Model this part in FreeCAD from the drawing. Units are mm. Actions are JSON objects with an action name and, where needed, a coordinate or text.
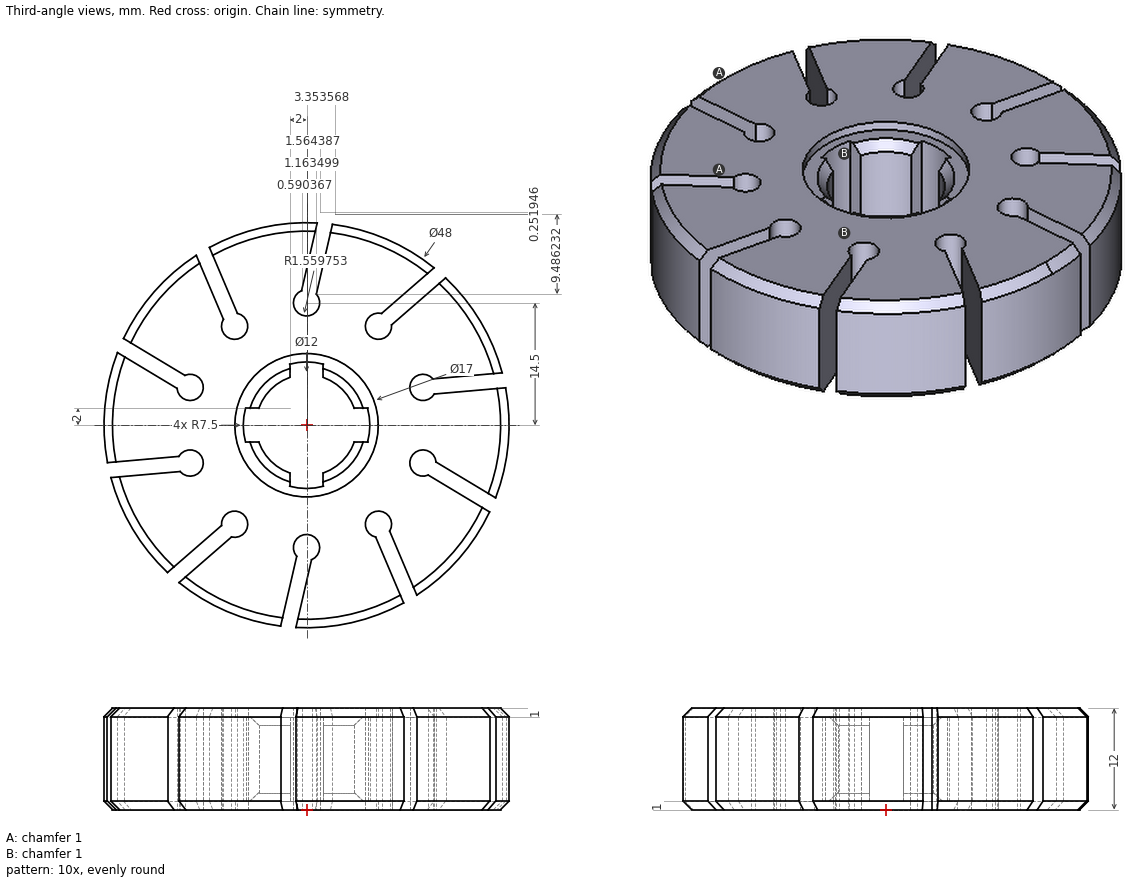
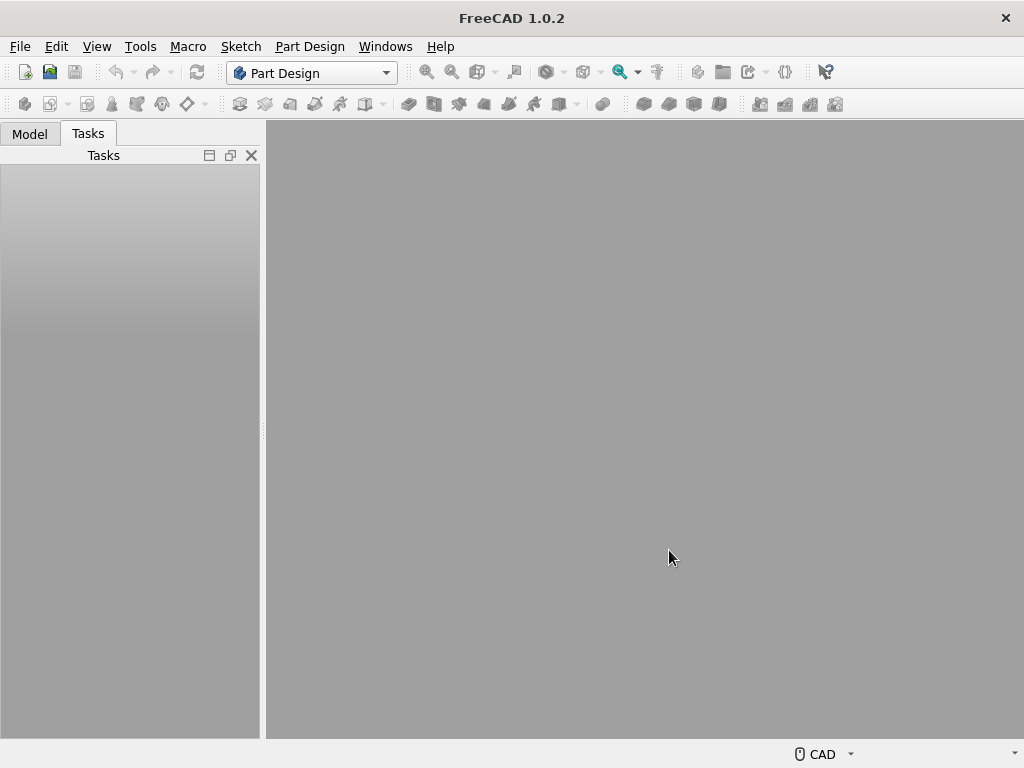
{"action": "left_click", "coordinate": [25, 72]}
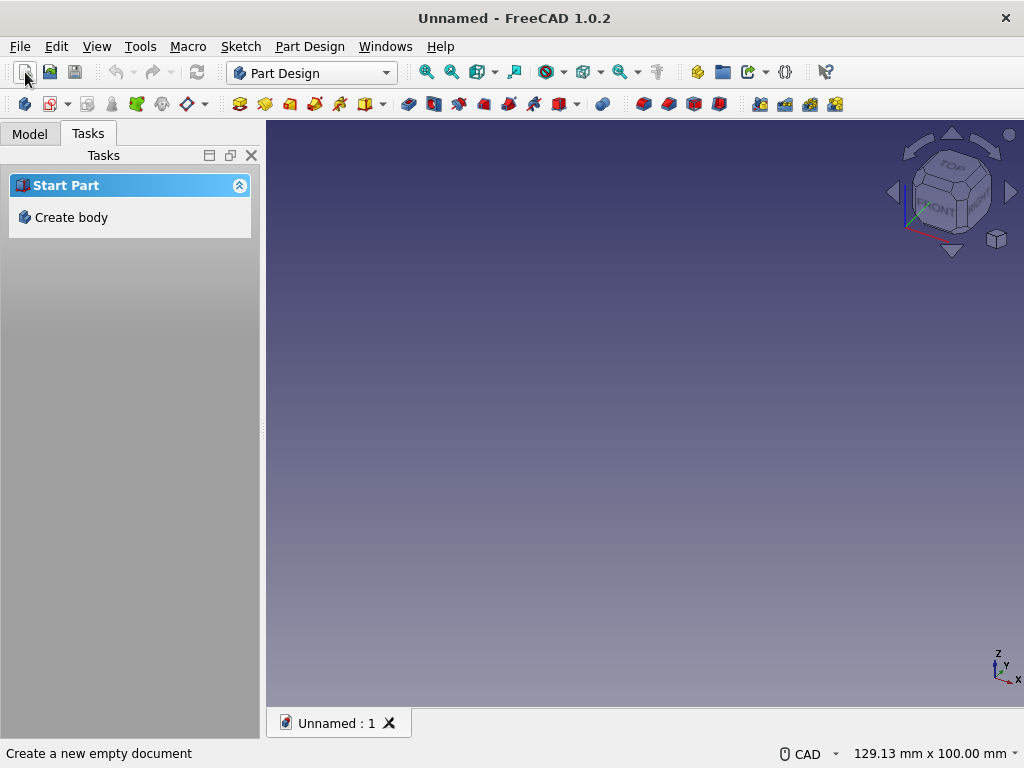
{"action": "left_click", "coordinate": [50, 104]}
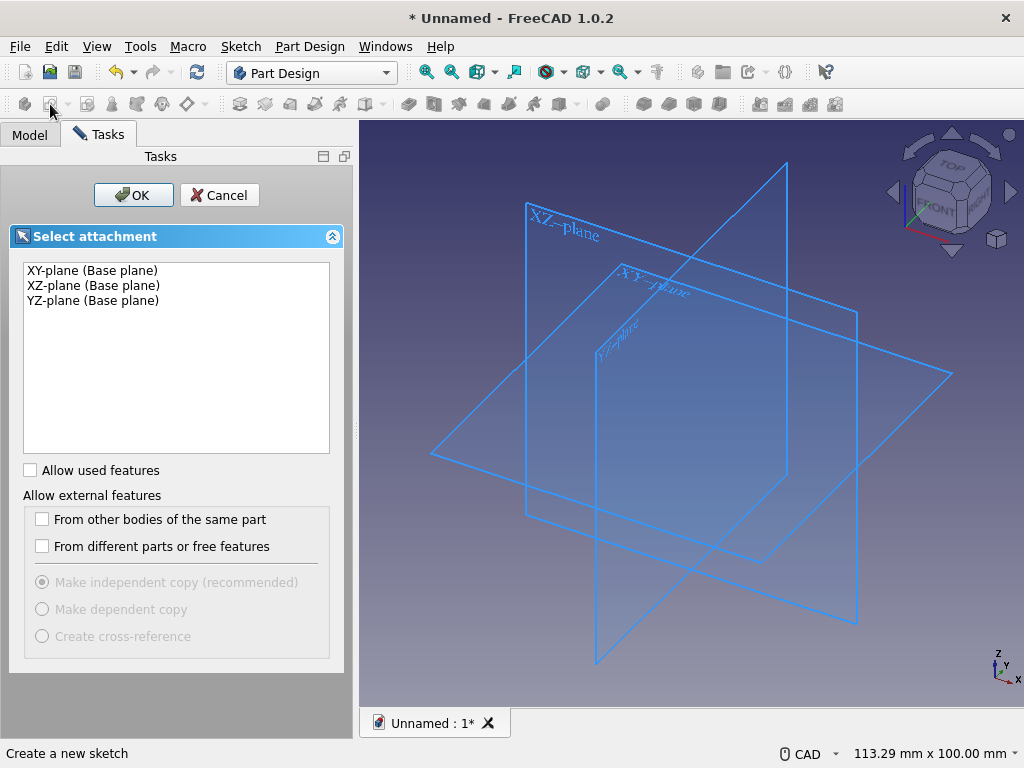
{"action": "left_click", "coordinate": [84, 270]}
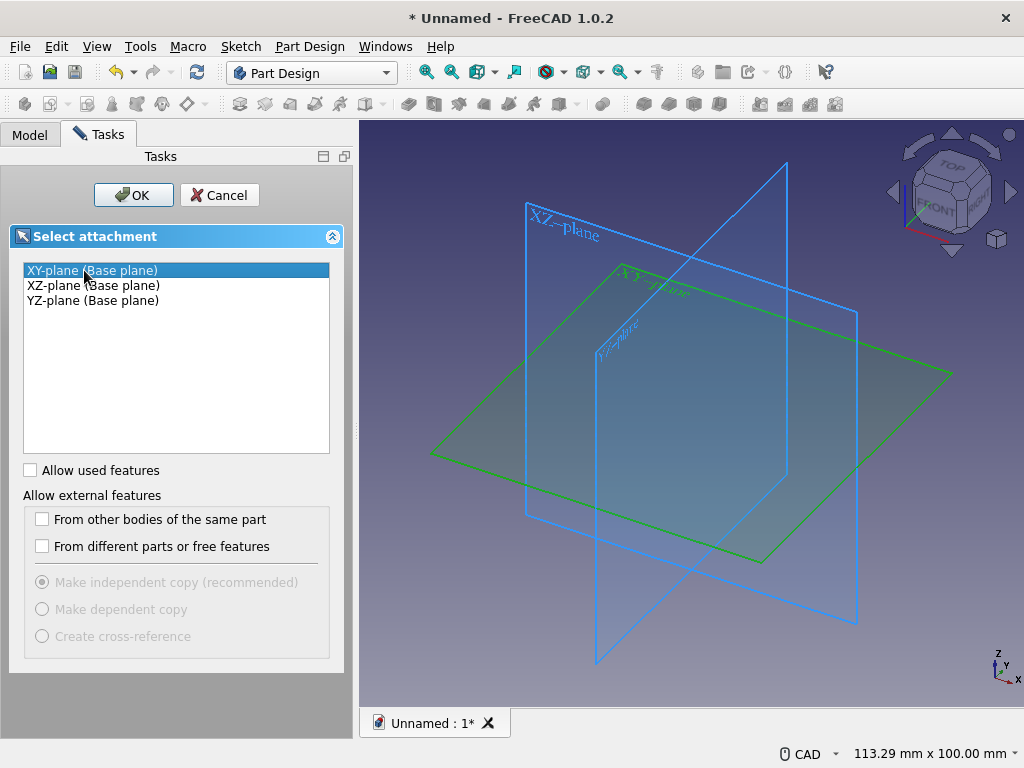
{"action": "left_click", "coordinate": [134, 195]}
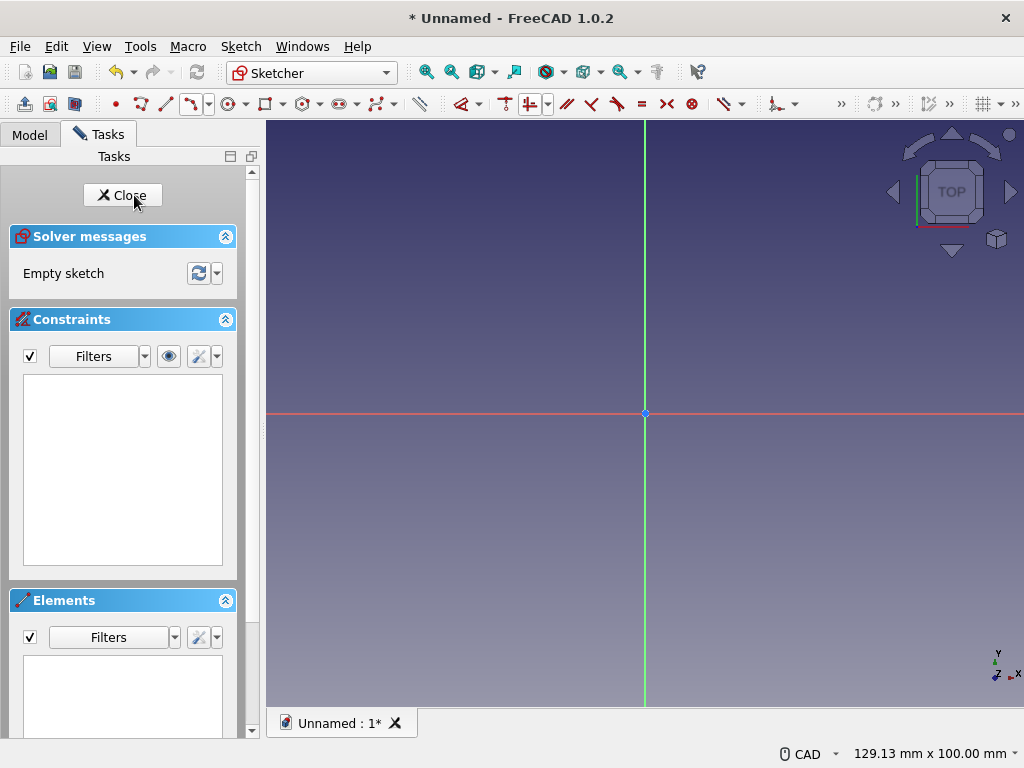
{"action": "left_click", "coordinate": [228, 104]}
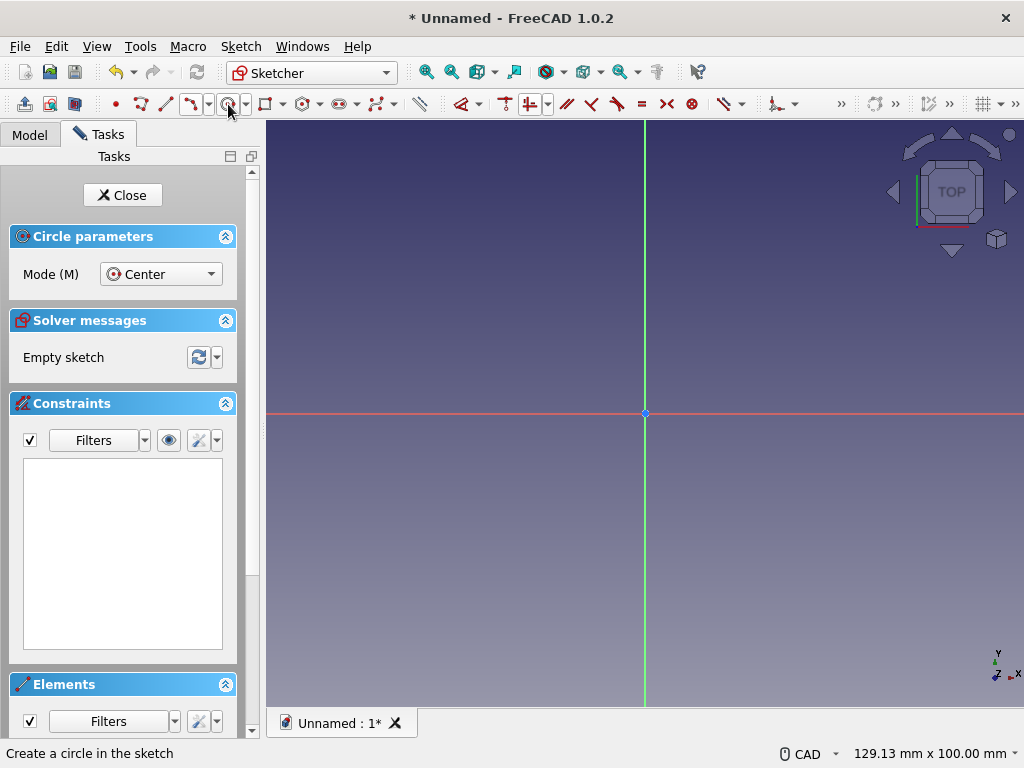
{"action": "left_click", "coordinate": [645, 414]}
{"action": "mouse_move", "coordinate": [745, 314]}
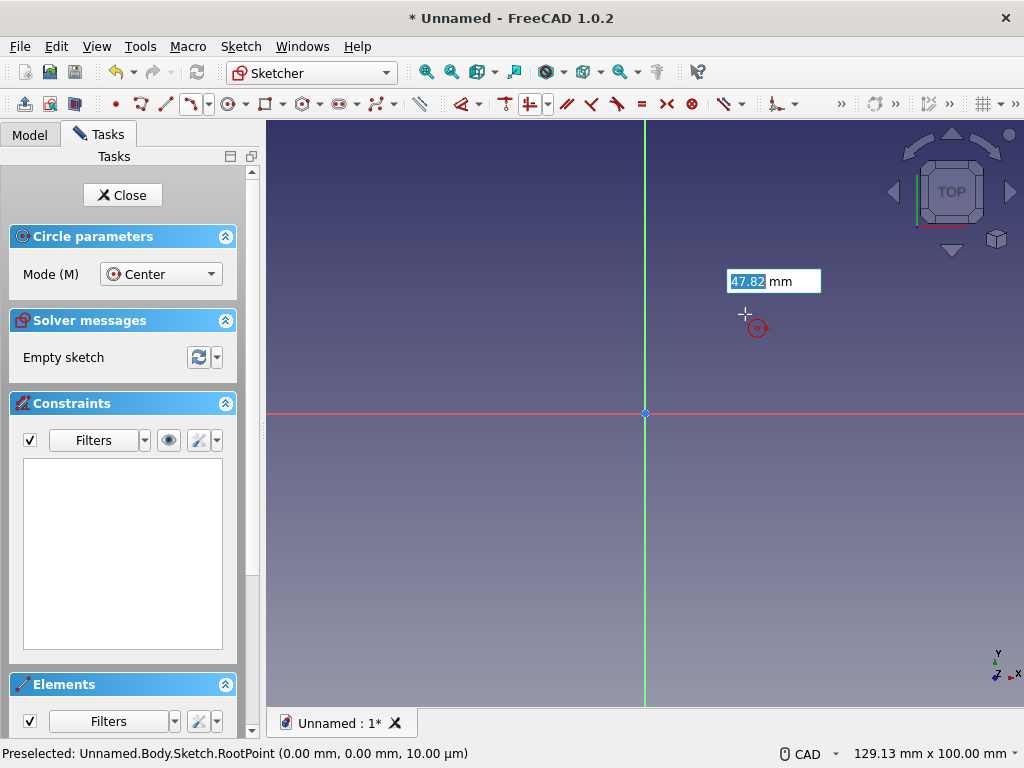
{"action": "type", "text": "48"}
{"action": "key", "text": "Return"}
{"action": "key", "text": "Escape"}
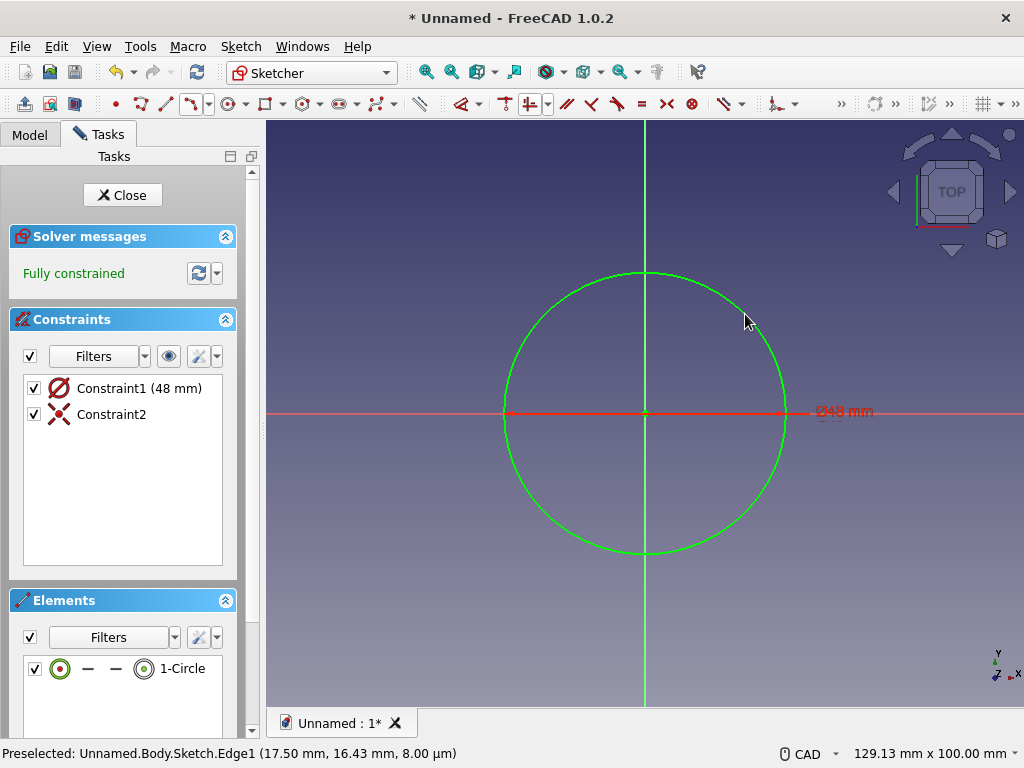
{"action": "left_click", "coordinate": [123, 195]}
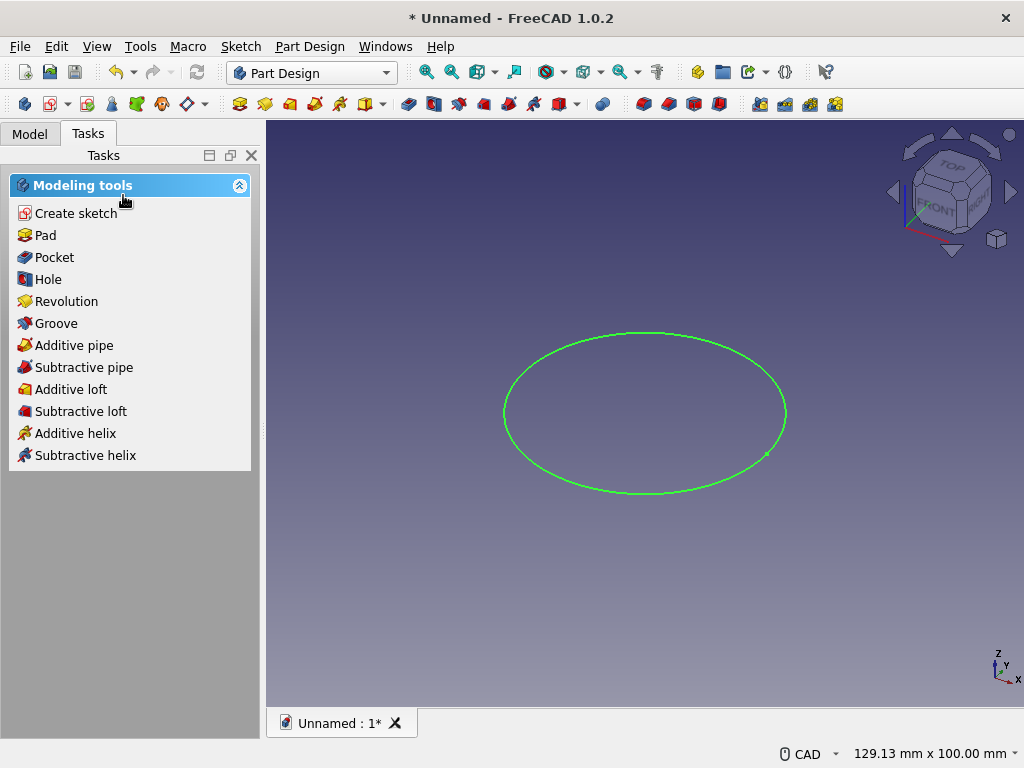
{"action": "left_click", "coordinate": [240, 104]}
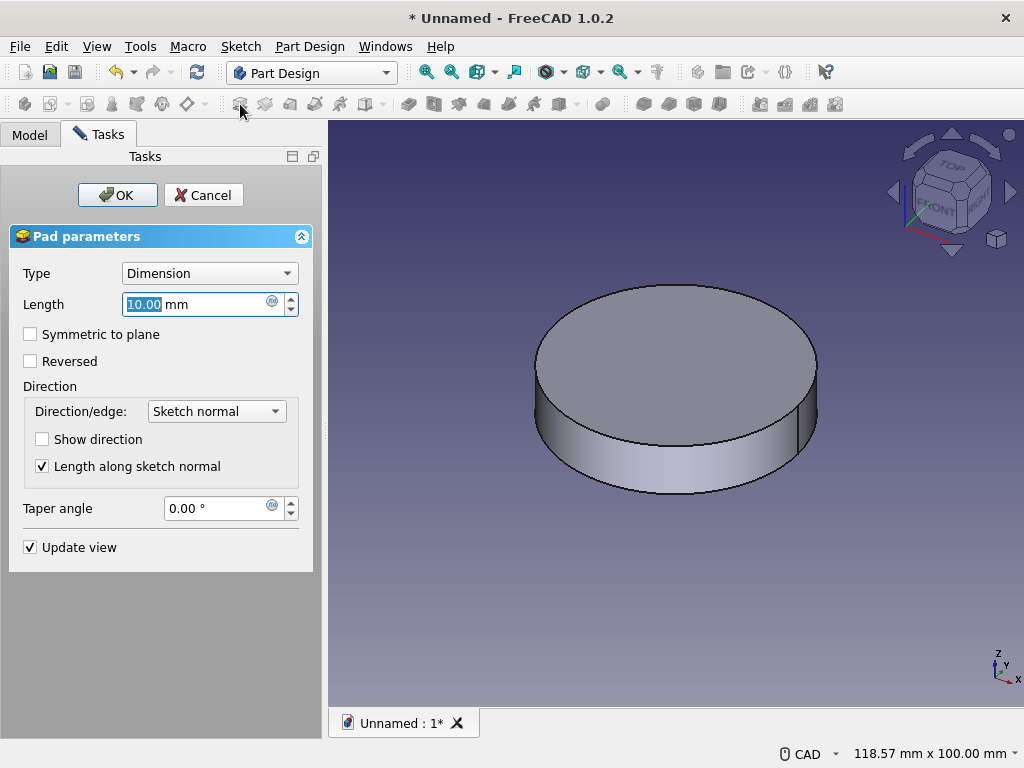
{"action": "type", "text": "12"}
{"action": "key", "text": "Tab"}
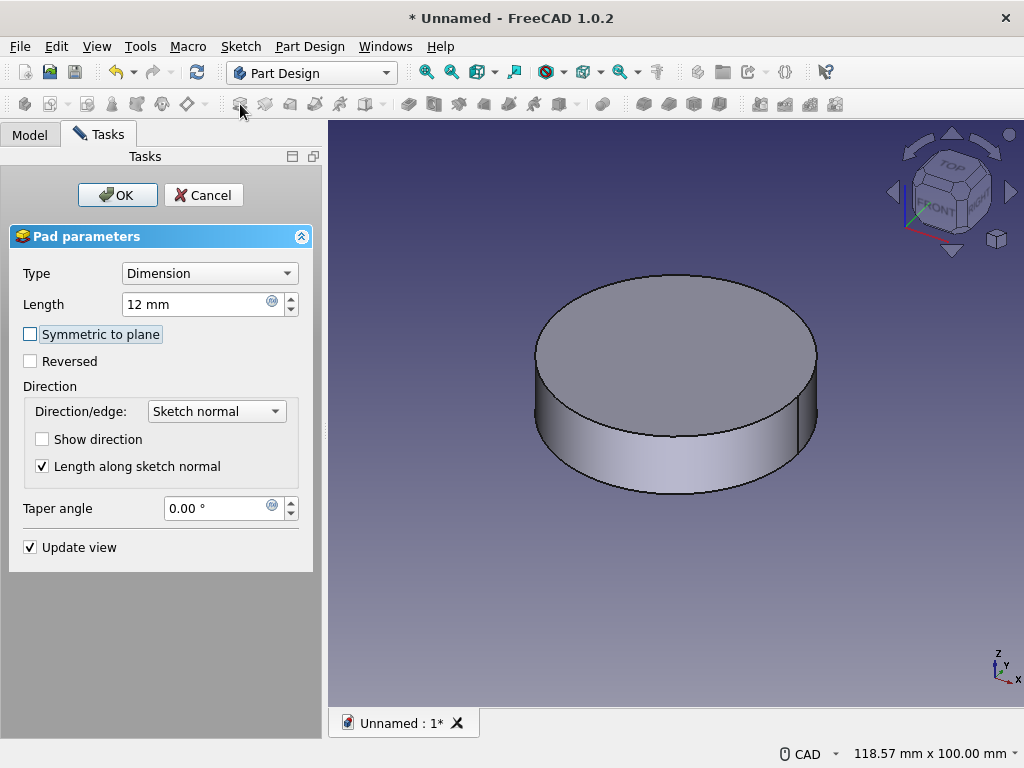
{"action": "left_click", "coordinate": [118, 195]}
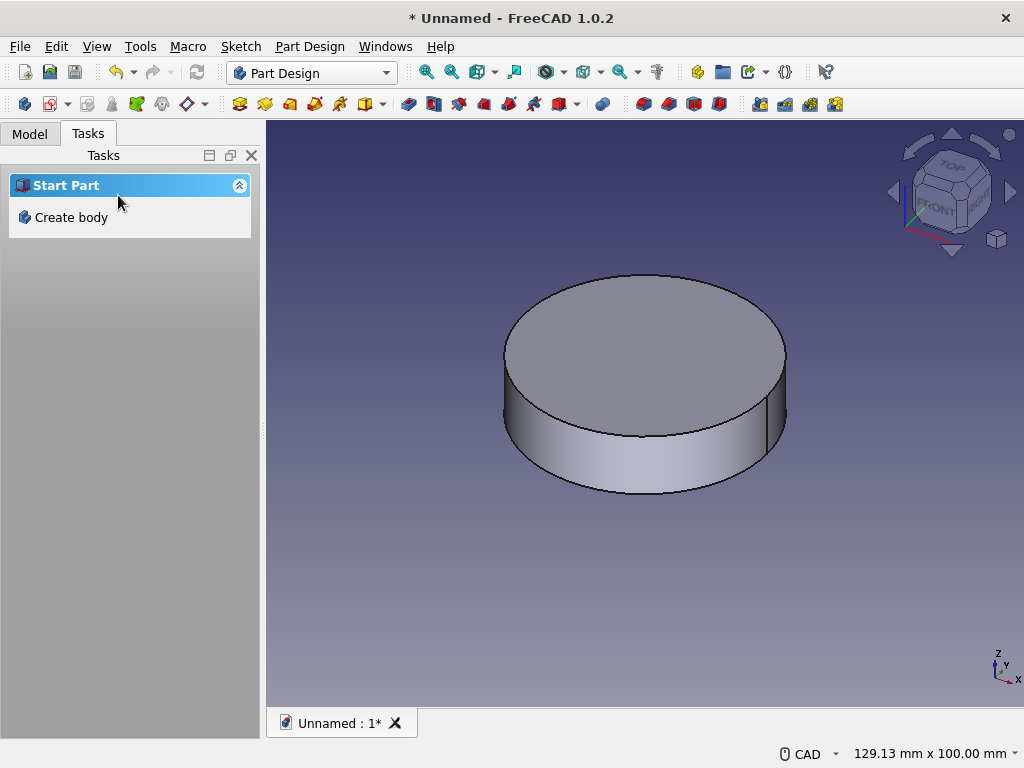
{"action": "left_click", "coordinate": [505, 363]}